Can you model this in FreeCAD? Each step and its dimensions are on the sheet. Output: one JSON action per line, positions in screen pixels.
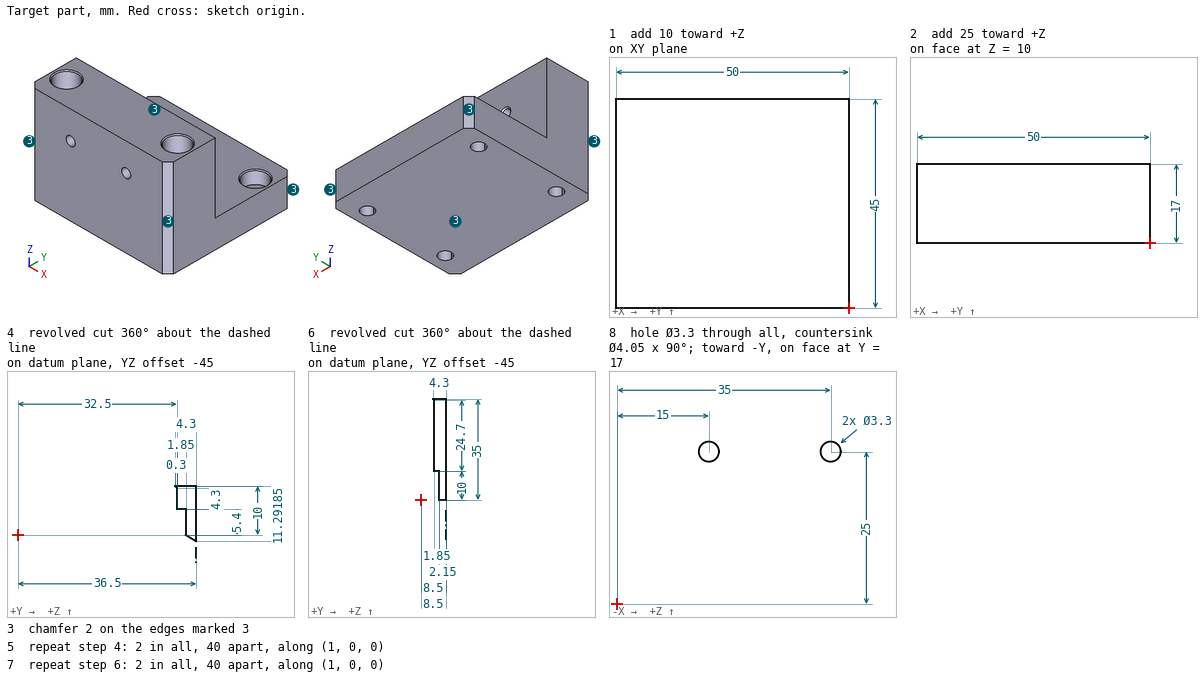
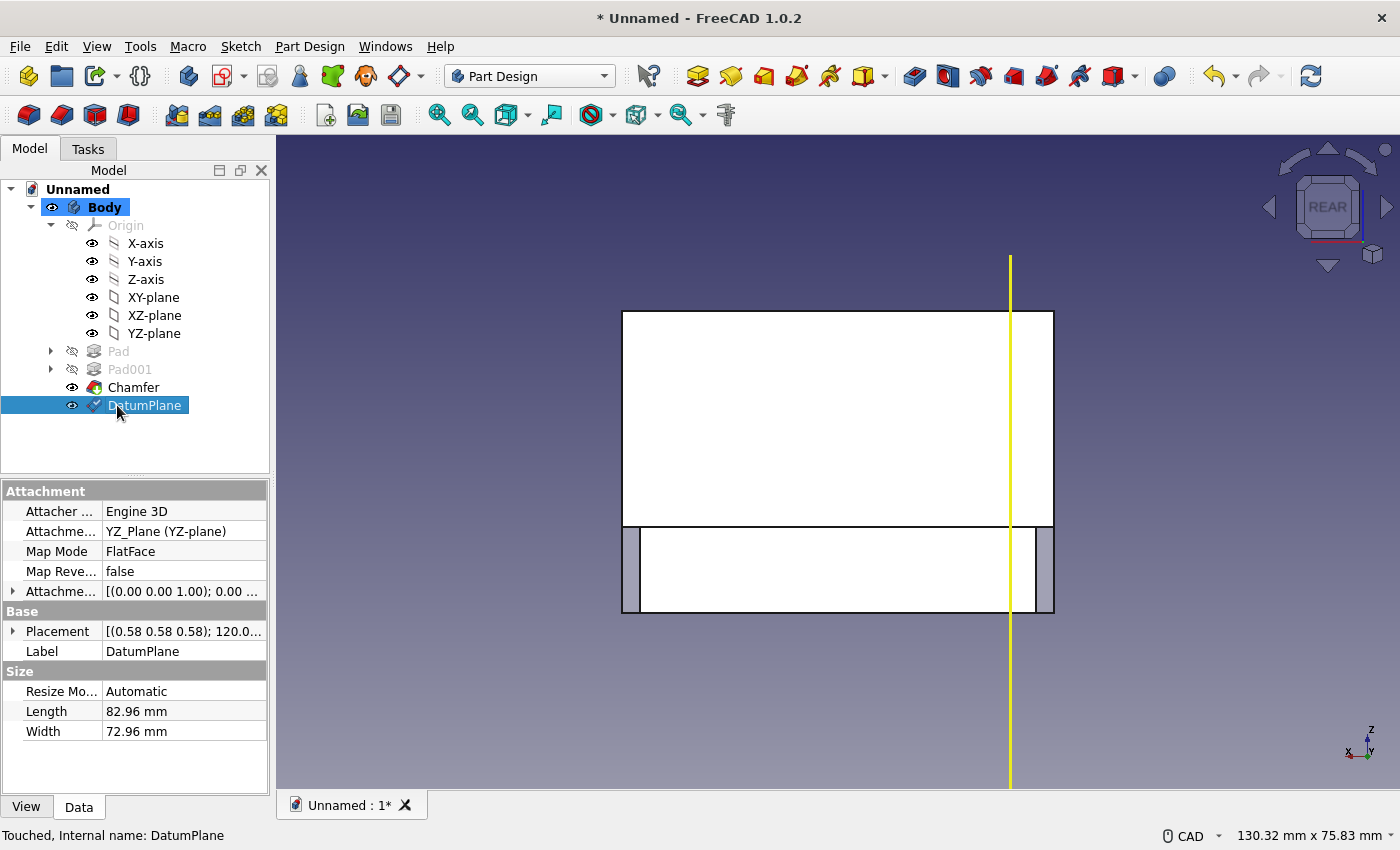
{"action": "left_click", "coordinate": [222, 76]}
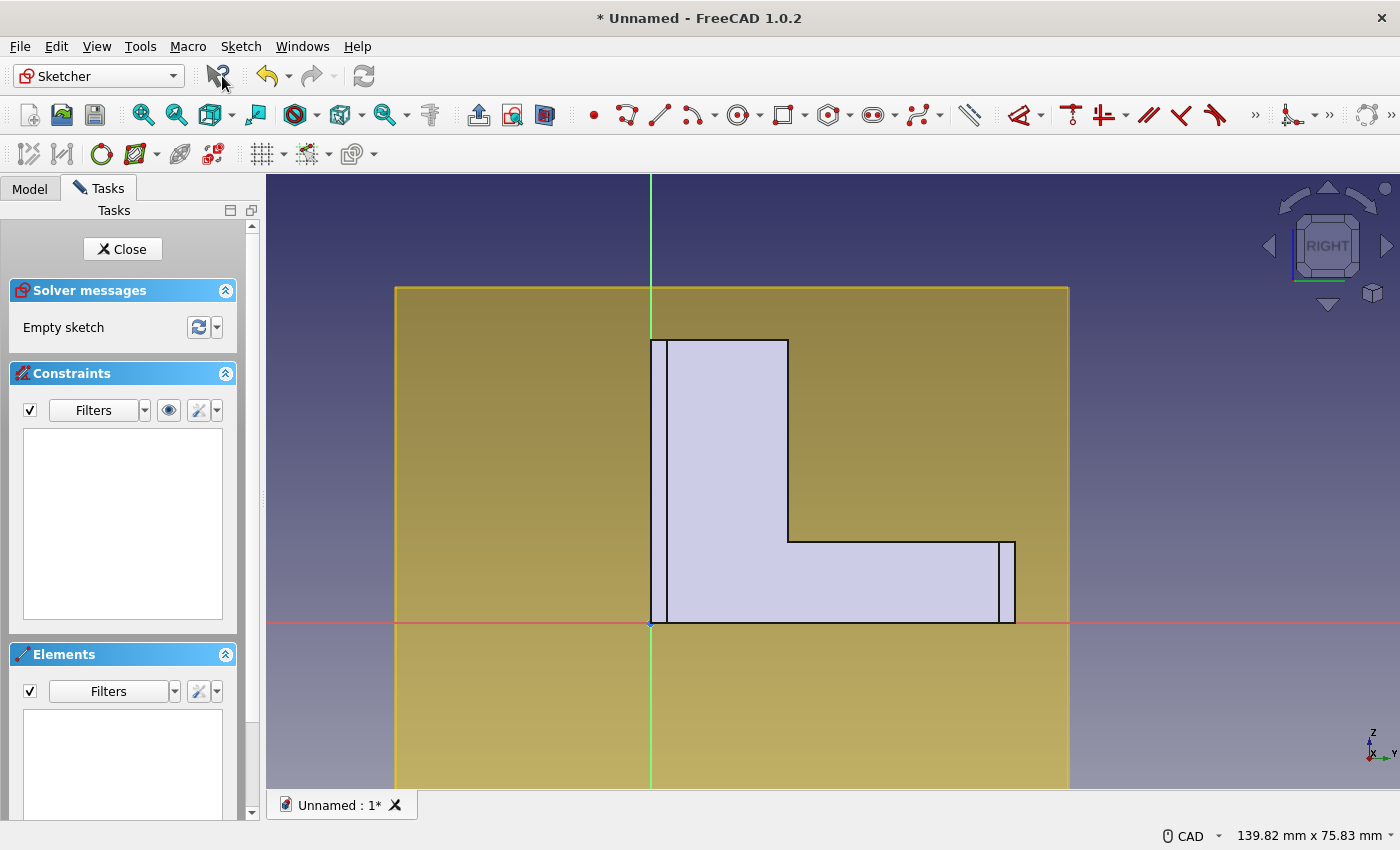
{"action": "left_click", "coordinate": [545, 116]}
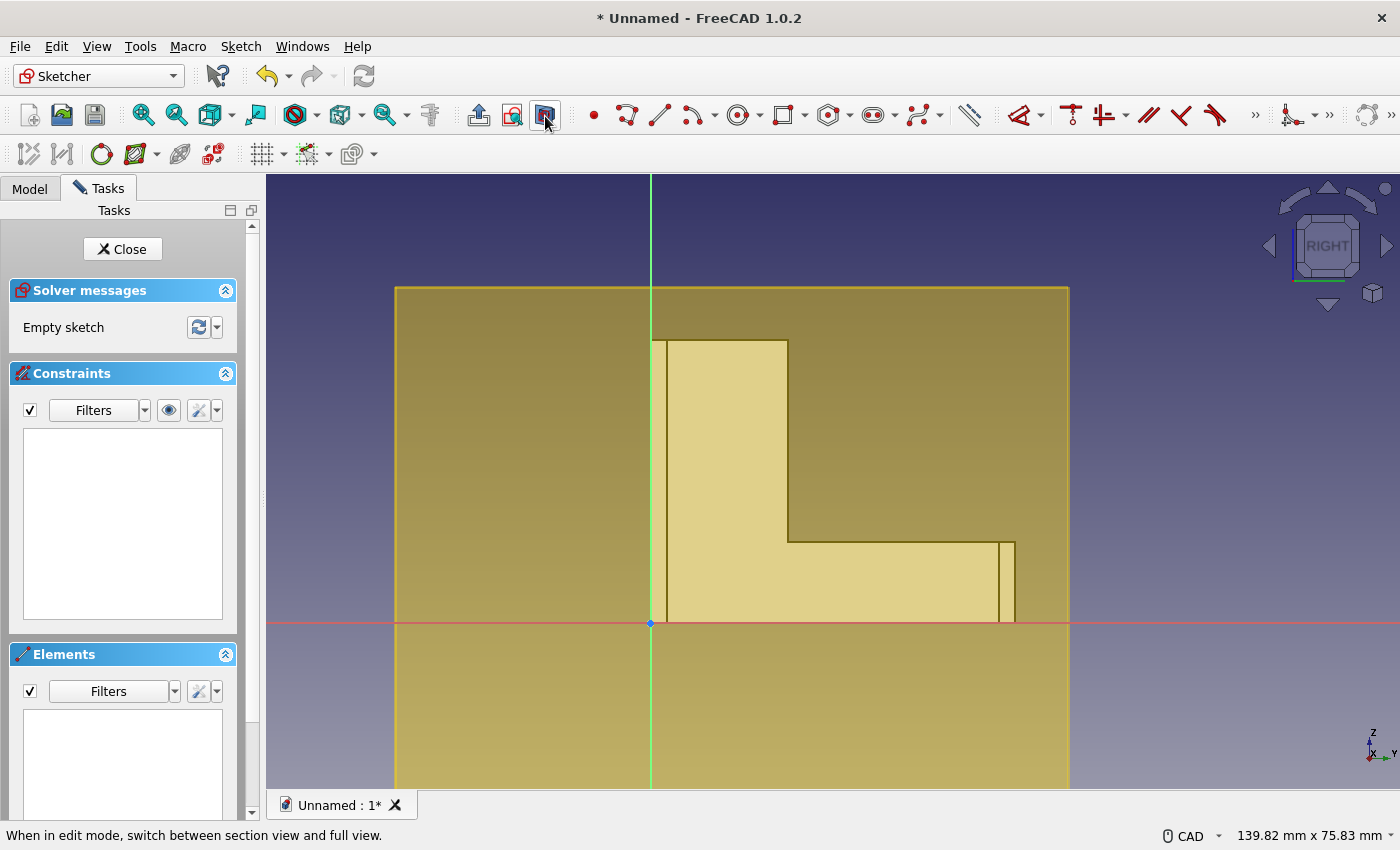
{"action": "scroll", "coordinate": [826, 708], "scroll_direction": "up", "scroll_amount": 4}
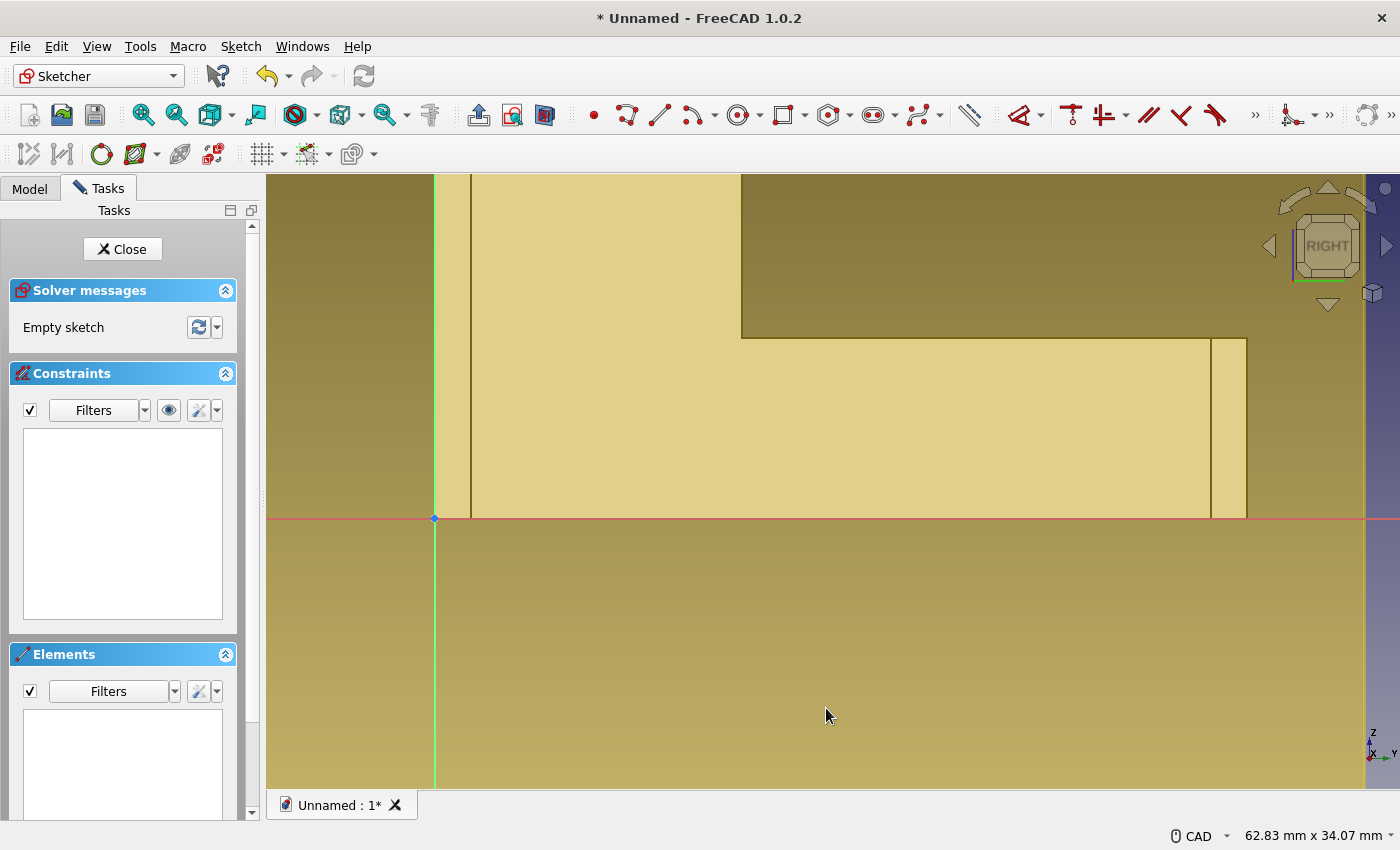
{"action": "key", "text": "g m"}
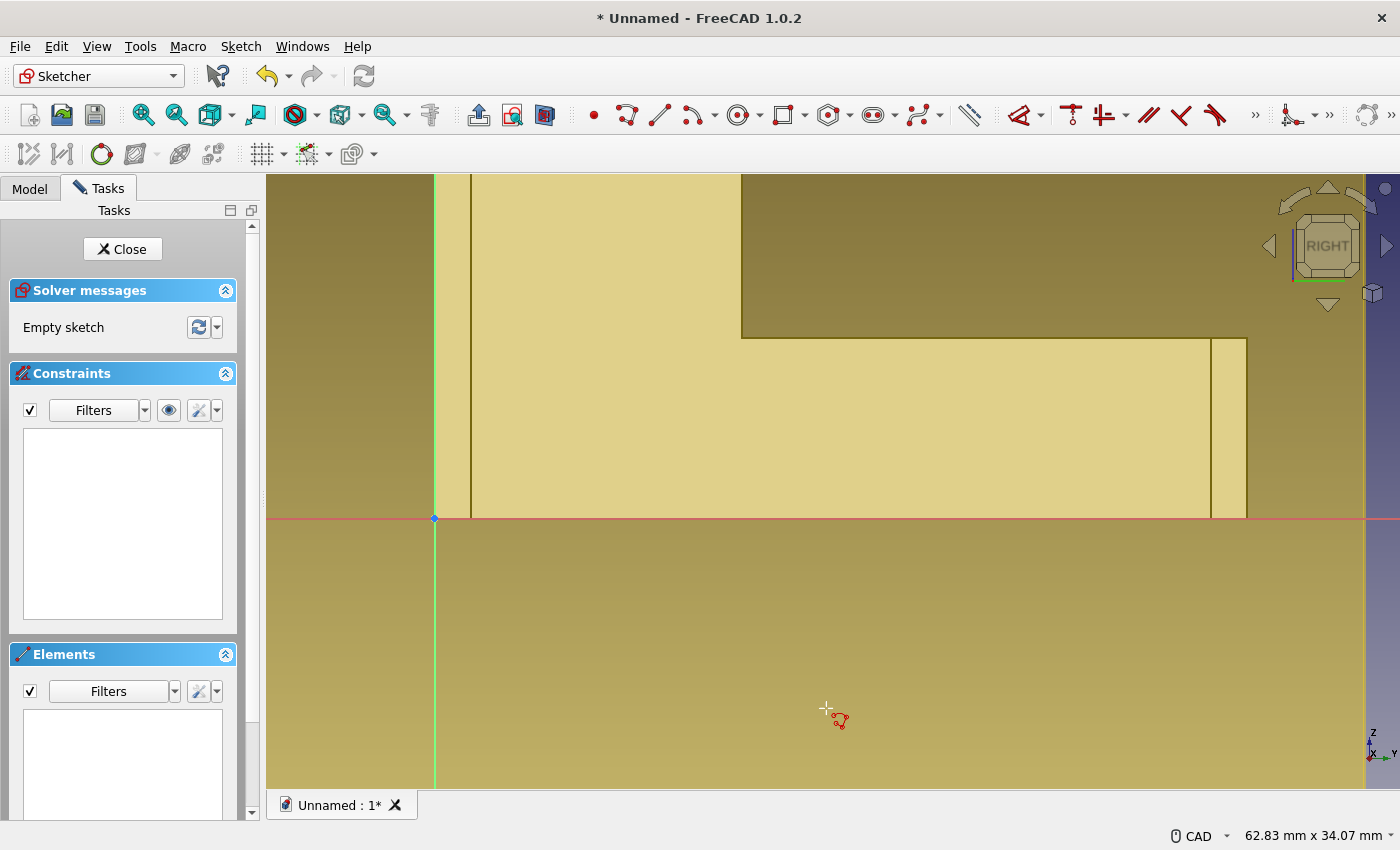
{"action": "left_click", "coordinate": [1021, 421]}
{"action": "left_click", "coordinate": [1055, 421]}
{"action": "left_click", "coordinate": [1055, 519]}
{"action": "left_click", "coordinate": [1094, 542]}
{"action": "left_click", "coordinate": [1094, 338]}
{"action": "left_click", "coordinate": [1016, 338]}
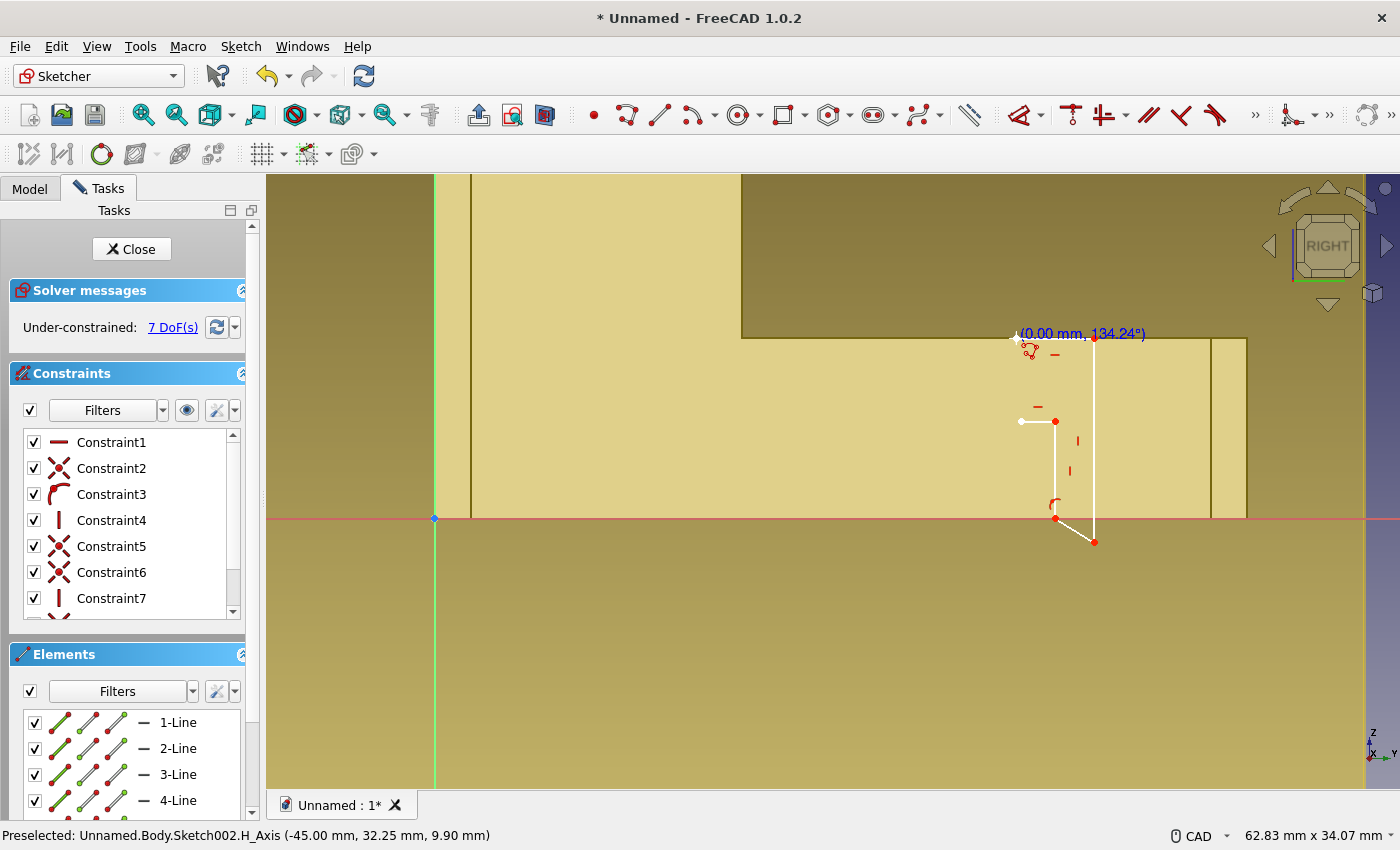
{"action": "scroll", "coordinate": [1021, 344], "scroll_direction": "up", "scroll_amount": 6}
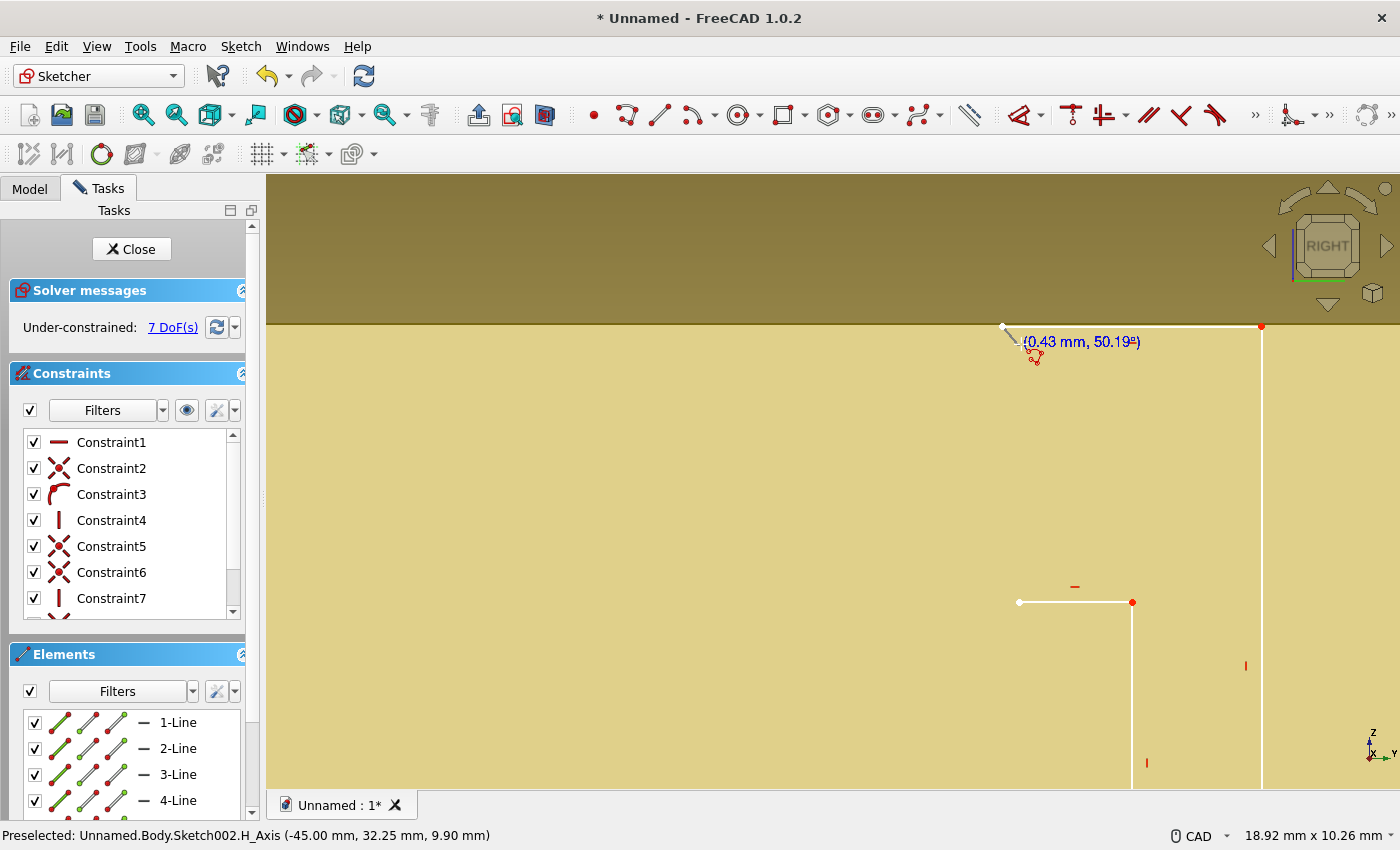
{"action": "left_click", "coordinate": [1021, 342]}
{"action": "left_click", "coordinate": [1019, 602]}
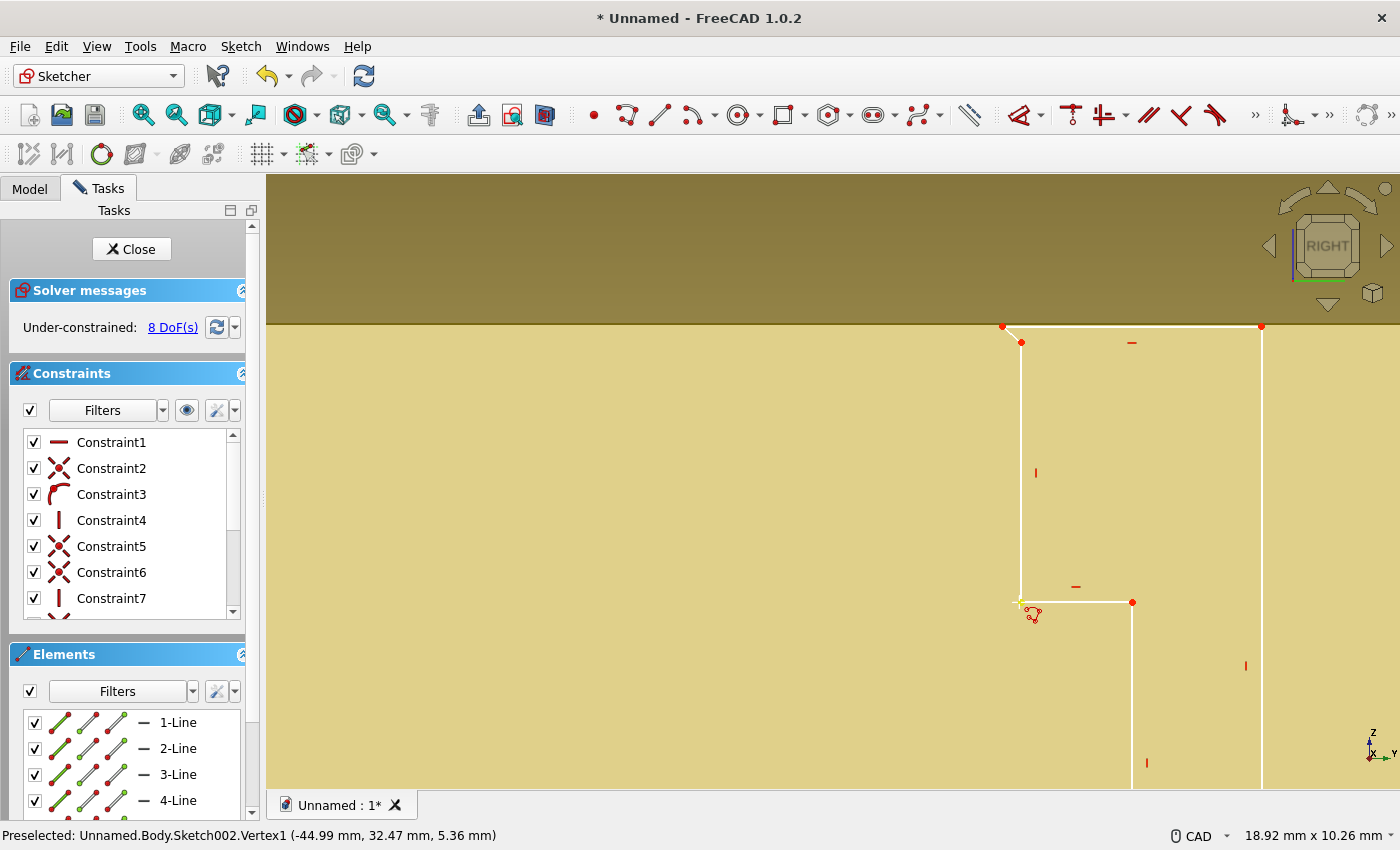
{"action": "key", "text": "g l"}